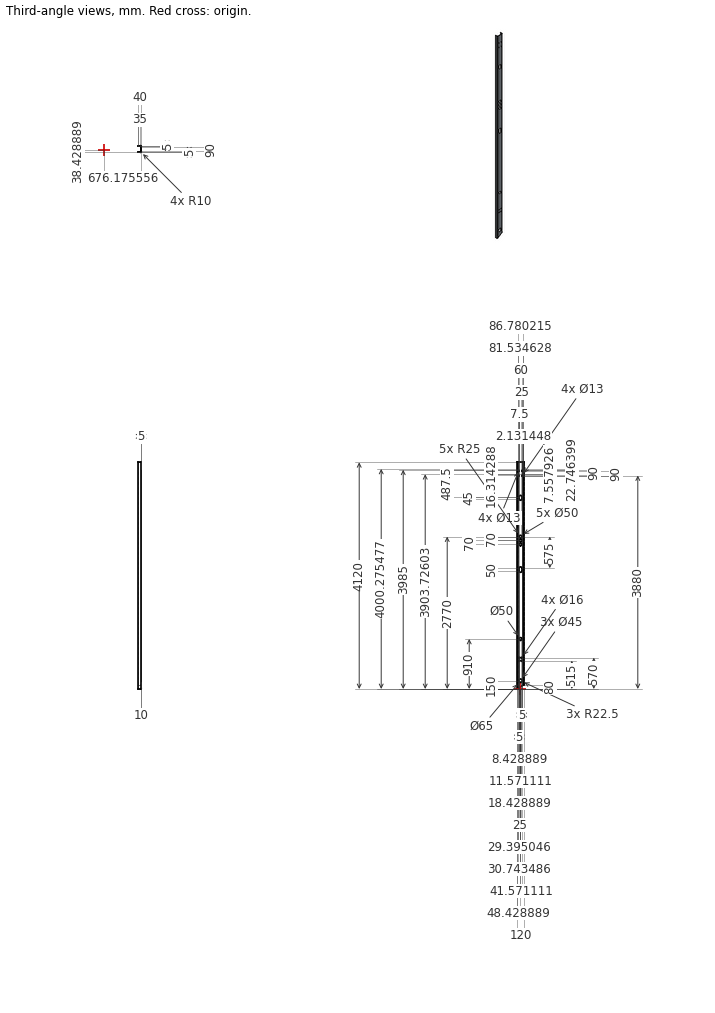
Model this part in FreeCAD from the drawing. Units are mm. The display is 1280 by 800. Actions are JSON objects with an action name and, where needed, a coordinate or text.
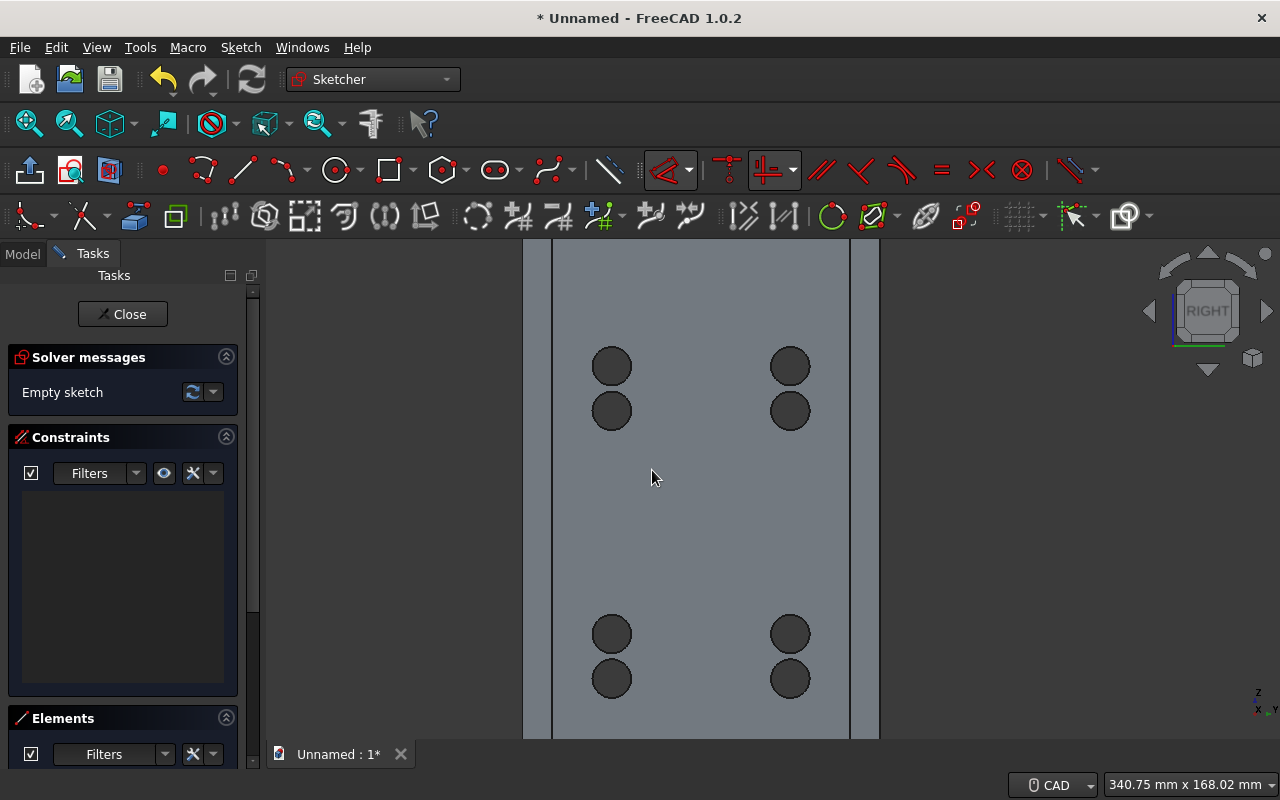
{"action": "key", "text": "g r"}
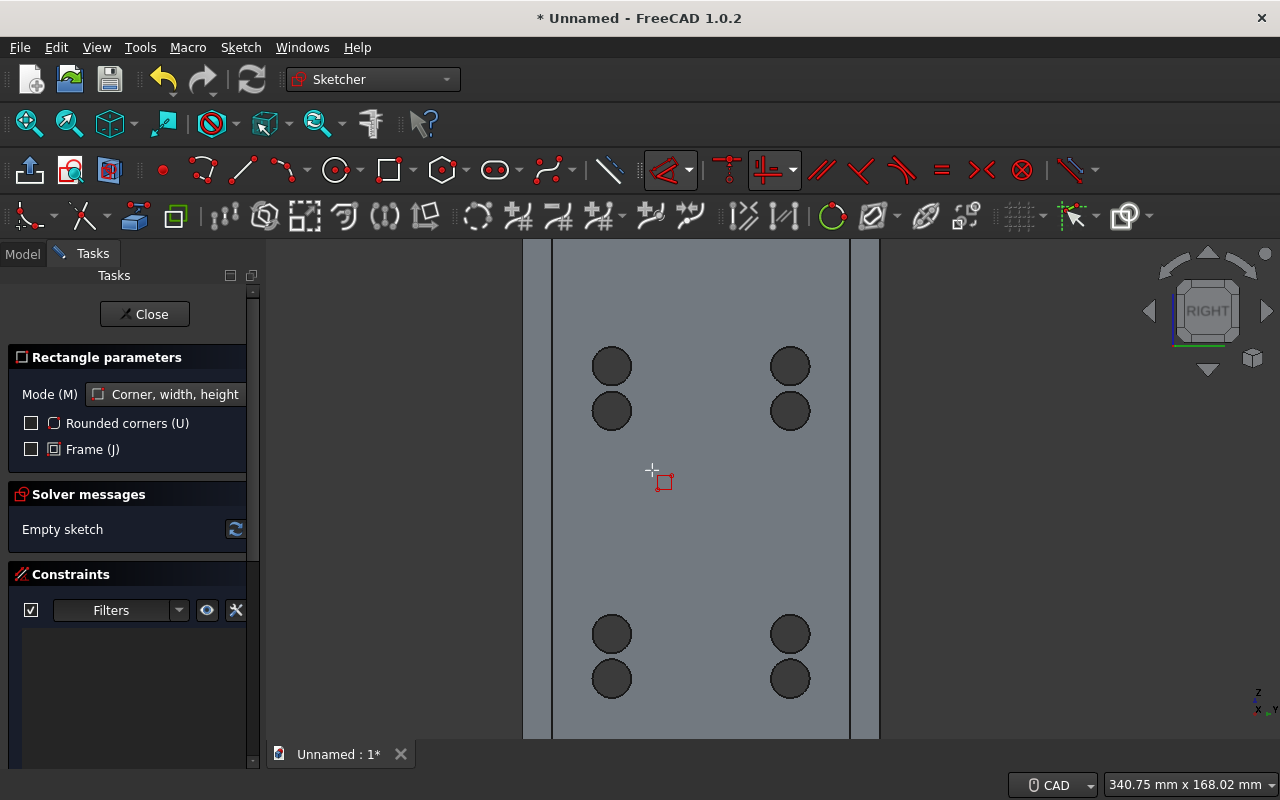
{"action": "left_click", "coordinate": [579, 321]}
{"action": "mouse_move", "coordinate": [822, 388]}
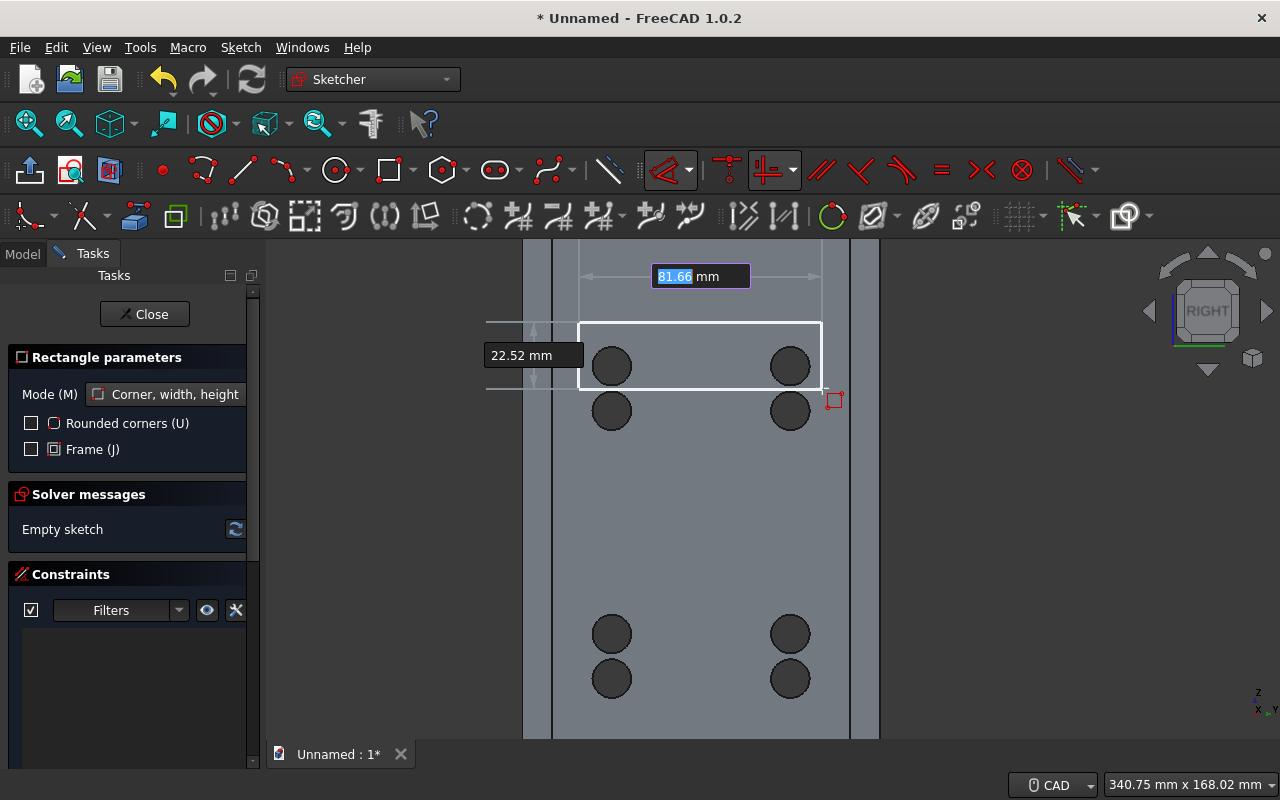
{"action": "type", "text": "81.534628"}
{"action": "key", "text": "Tab"}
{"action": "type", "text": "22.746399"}
{"action": "key", "text": "Return"}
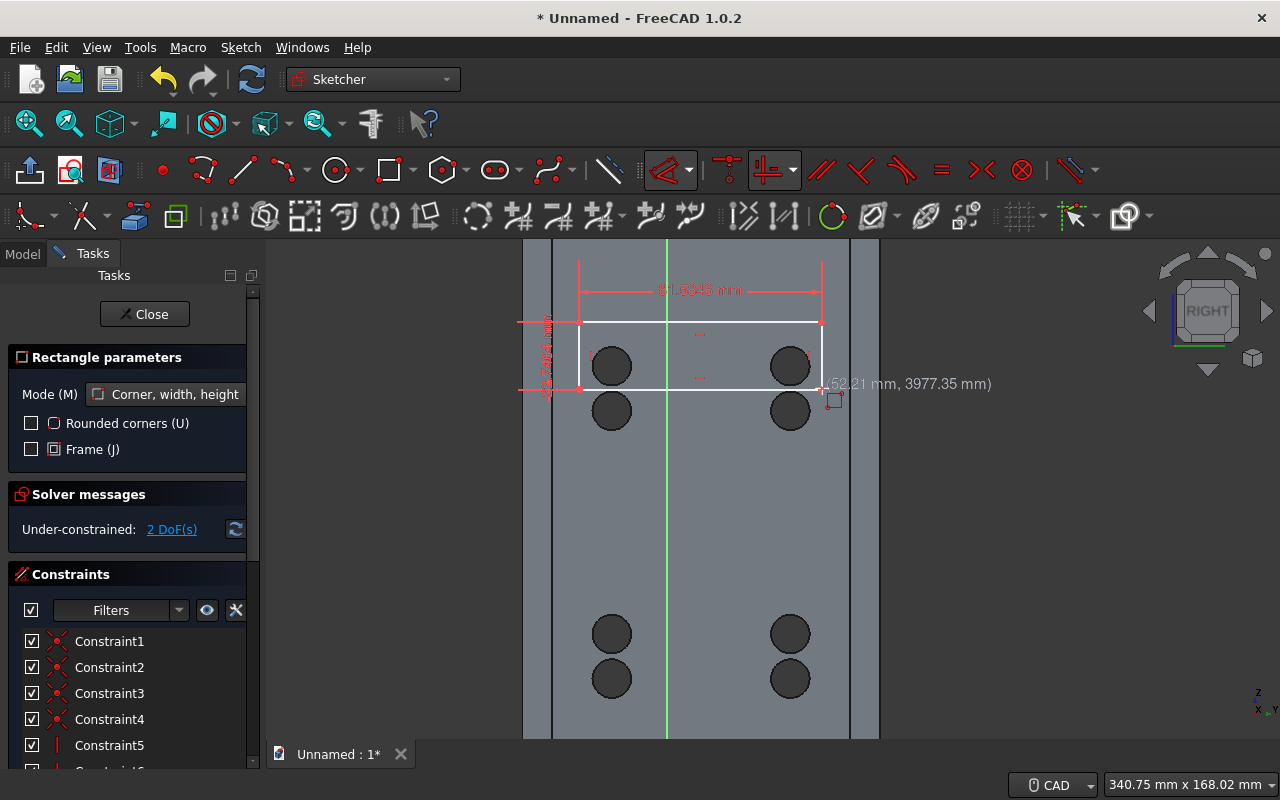
{"action": "key", "text": "g m"}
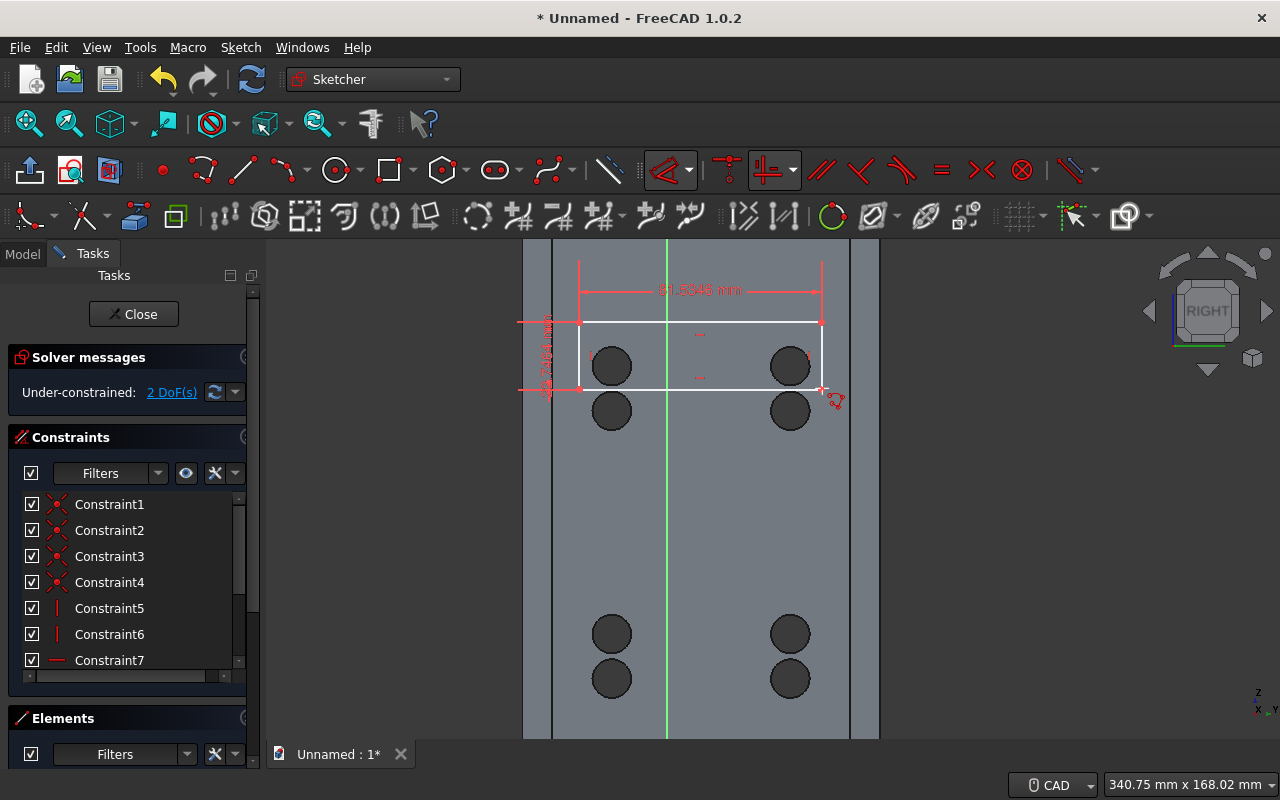
{"action": "left_click", "coordinate": [575, 657]}
{"action": "left_click", "coordinate": [833, 657]}
{"action": "left_click", "coordinate": [827, 586]}
{"action": "left_click", "coordinate": [575, 608]}
{"action": "left_click", "coordinate": [575, 658]}
{"action": "key", "text": "Escape"}
{"action": "key", "text": "Escape"}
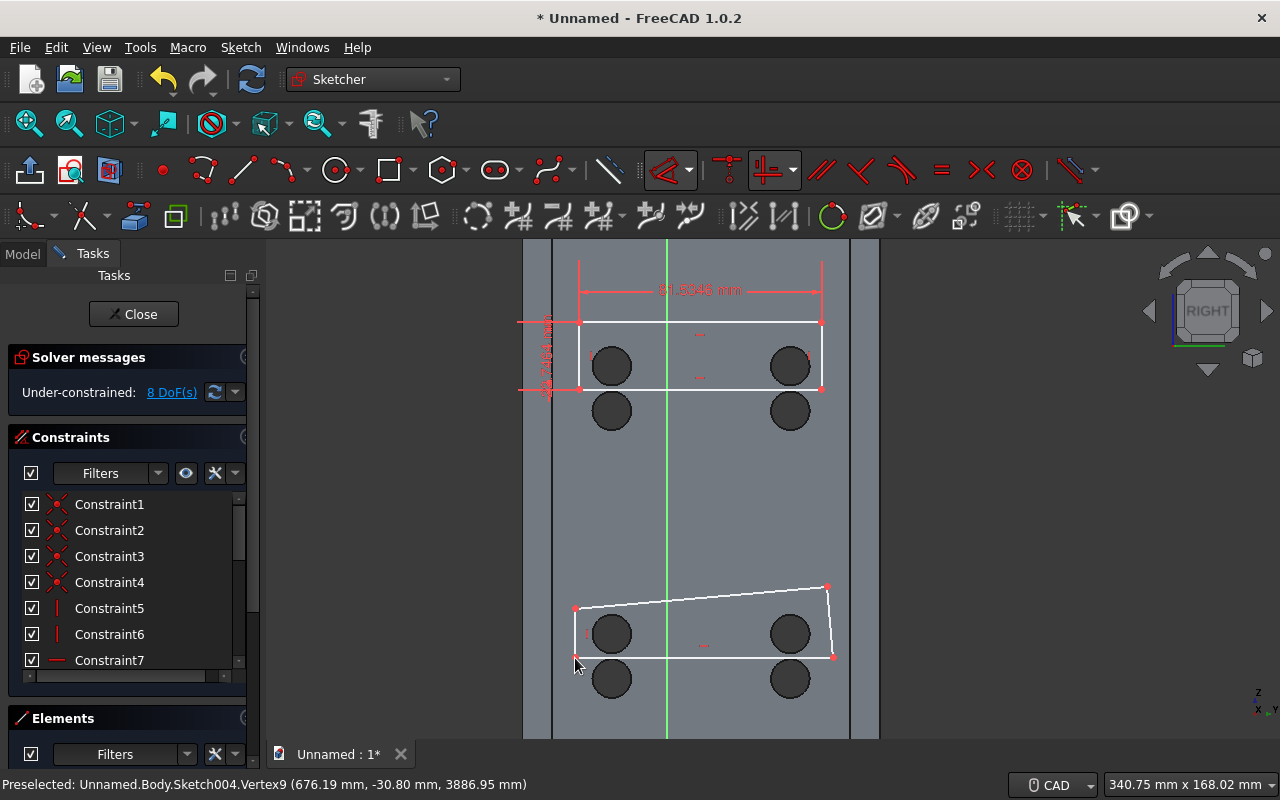
{"action": "left_click", "coordinate": [652, 658]}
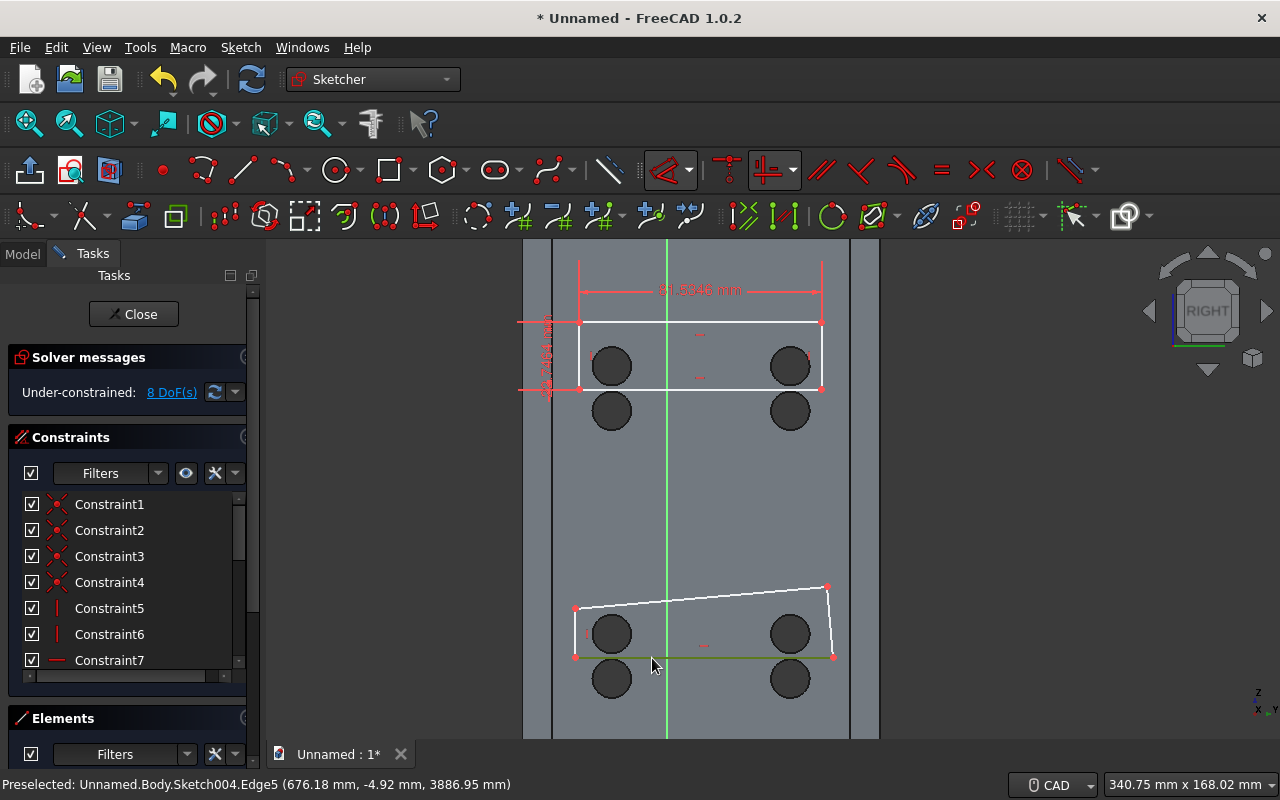
{"action": "key", "text": "l"}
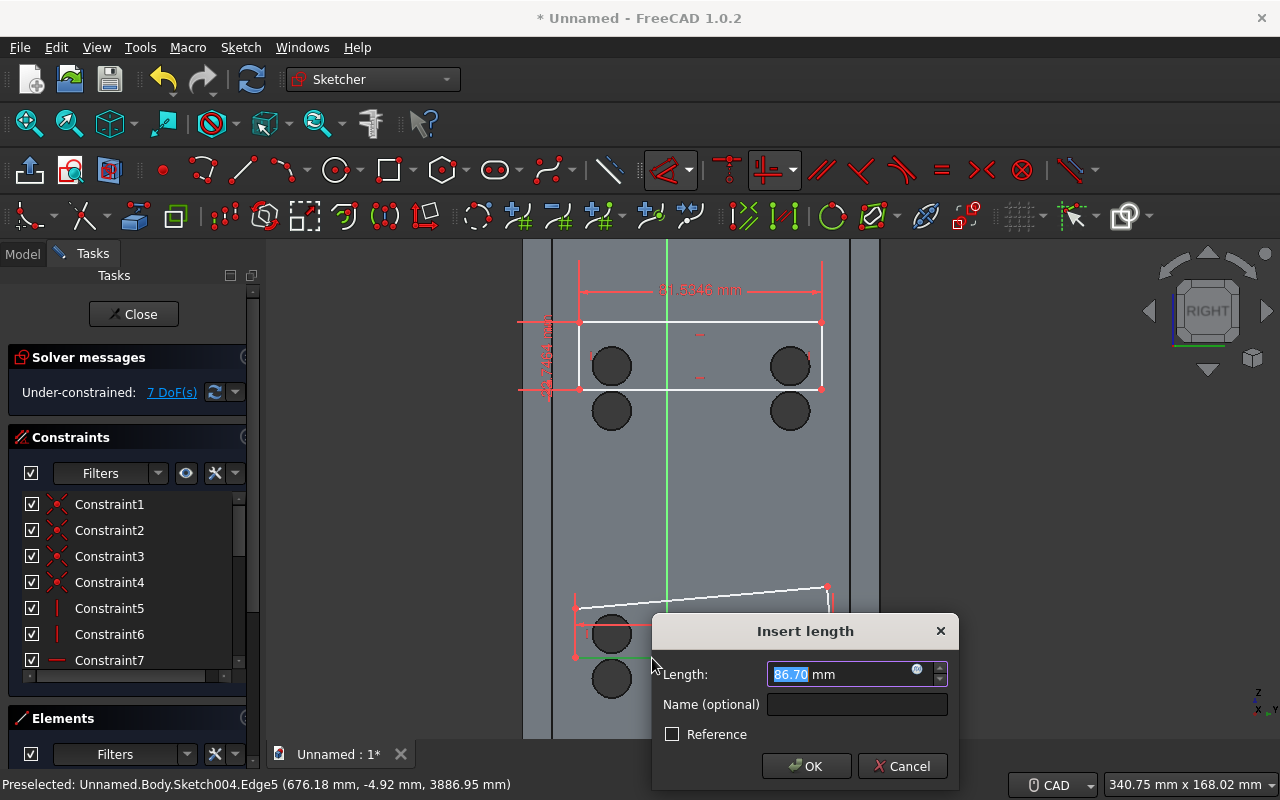
{"action": "type", "text": "86.780215"}
{"action": "key", "text": "Return"}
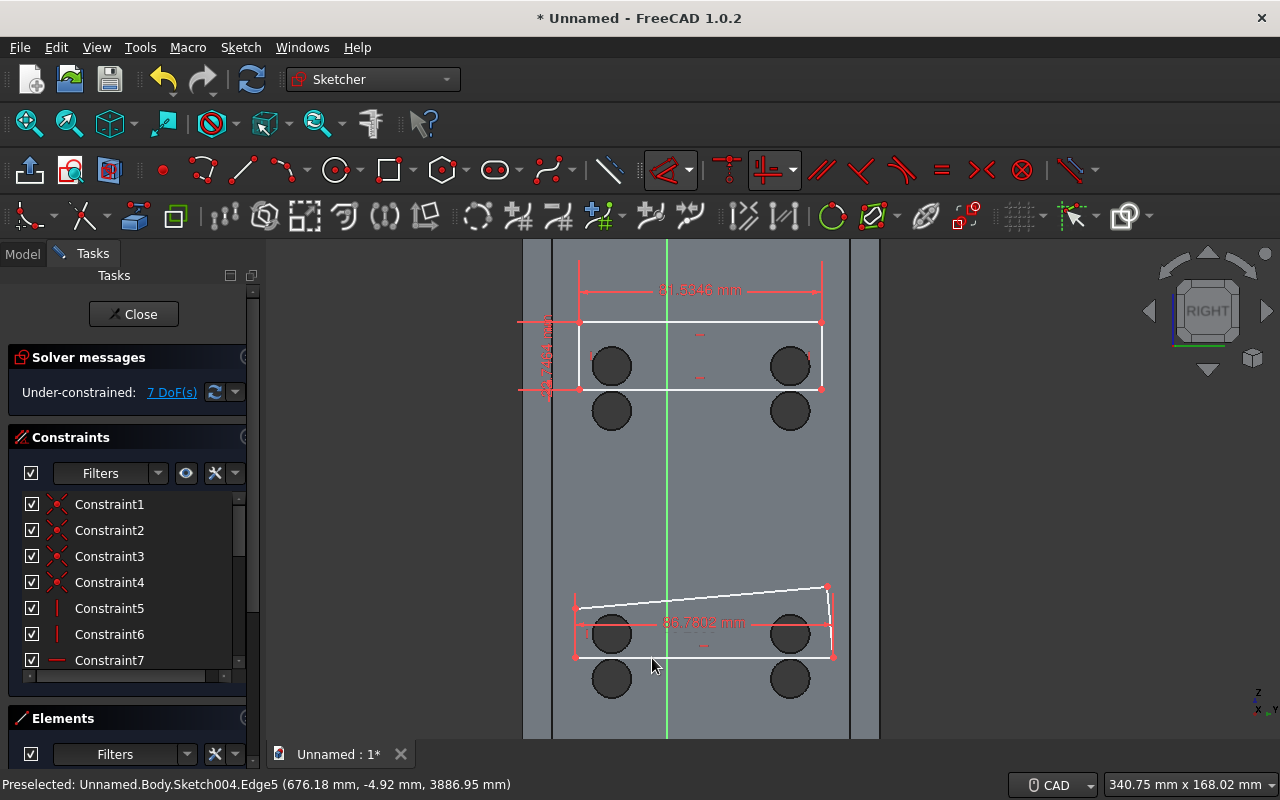
{"action": "left_click", "coordinate": [575, 624]}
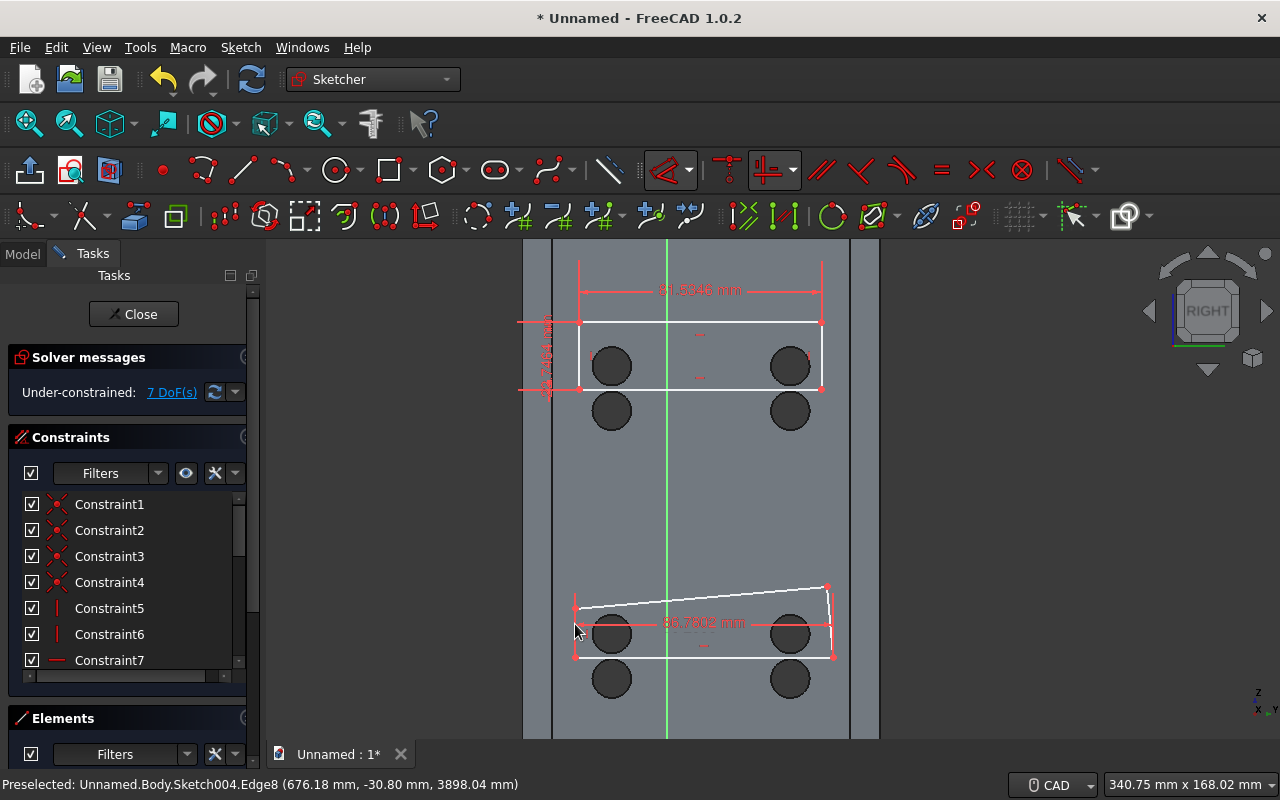
{"action": "key", "text": "i"}